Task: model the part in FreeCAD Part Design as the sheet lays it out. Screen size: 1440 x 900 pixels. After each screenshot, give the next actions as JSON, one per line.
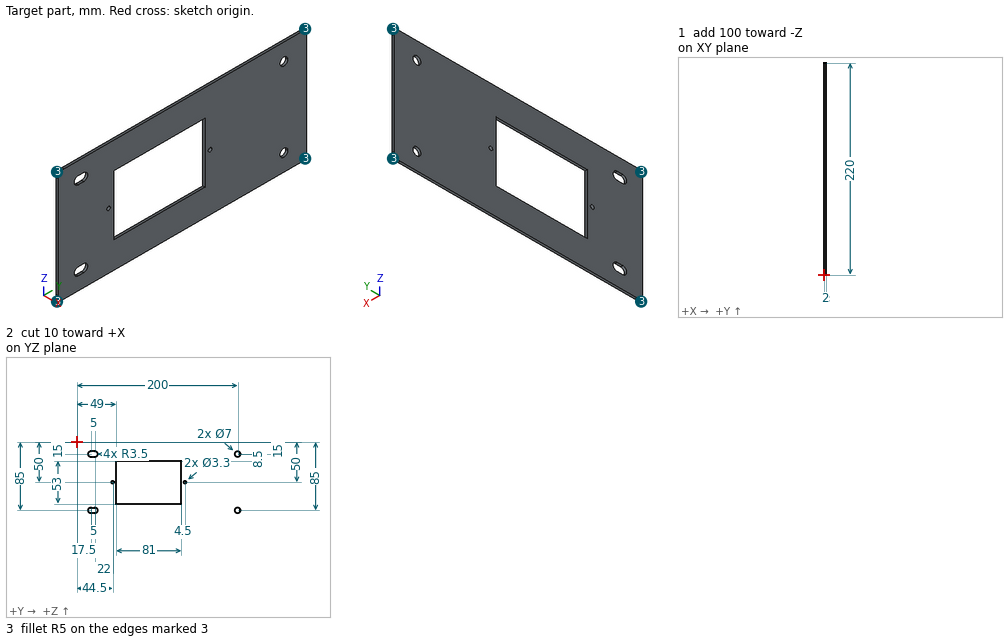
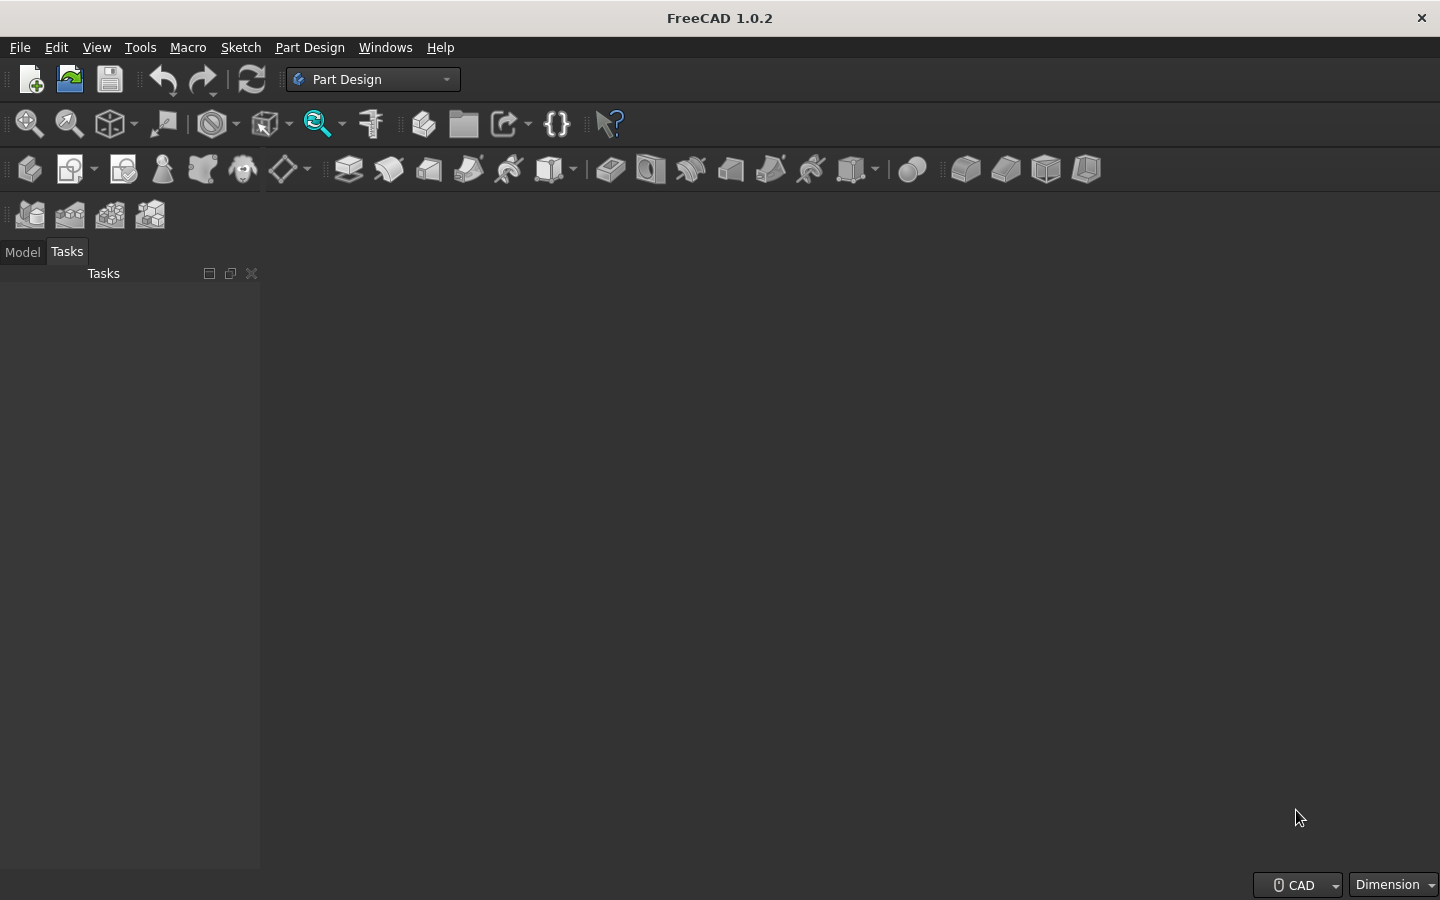
{"action": "left_click", "coordinate": [1024, 80]}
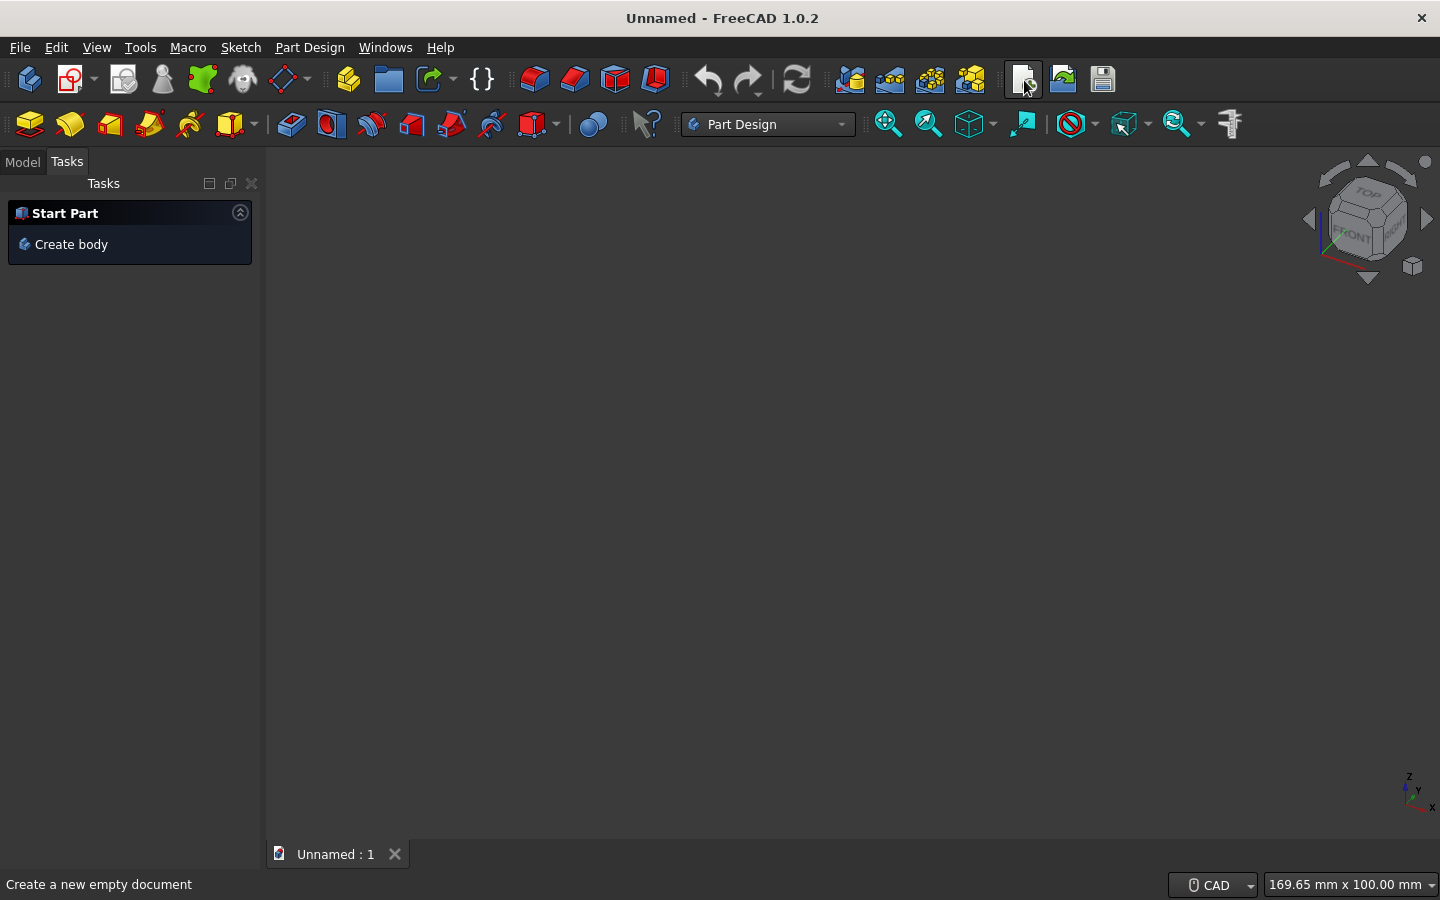
{"action": "left_click", "coordinate": [70, 80]}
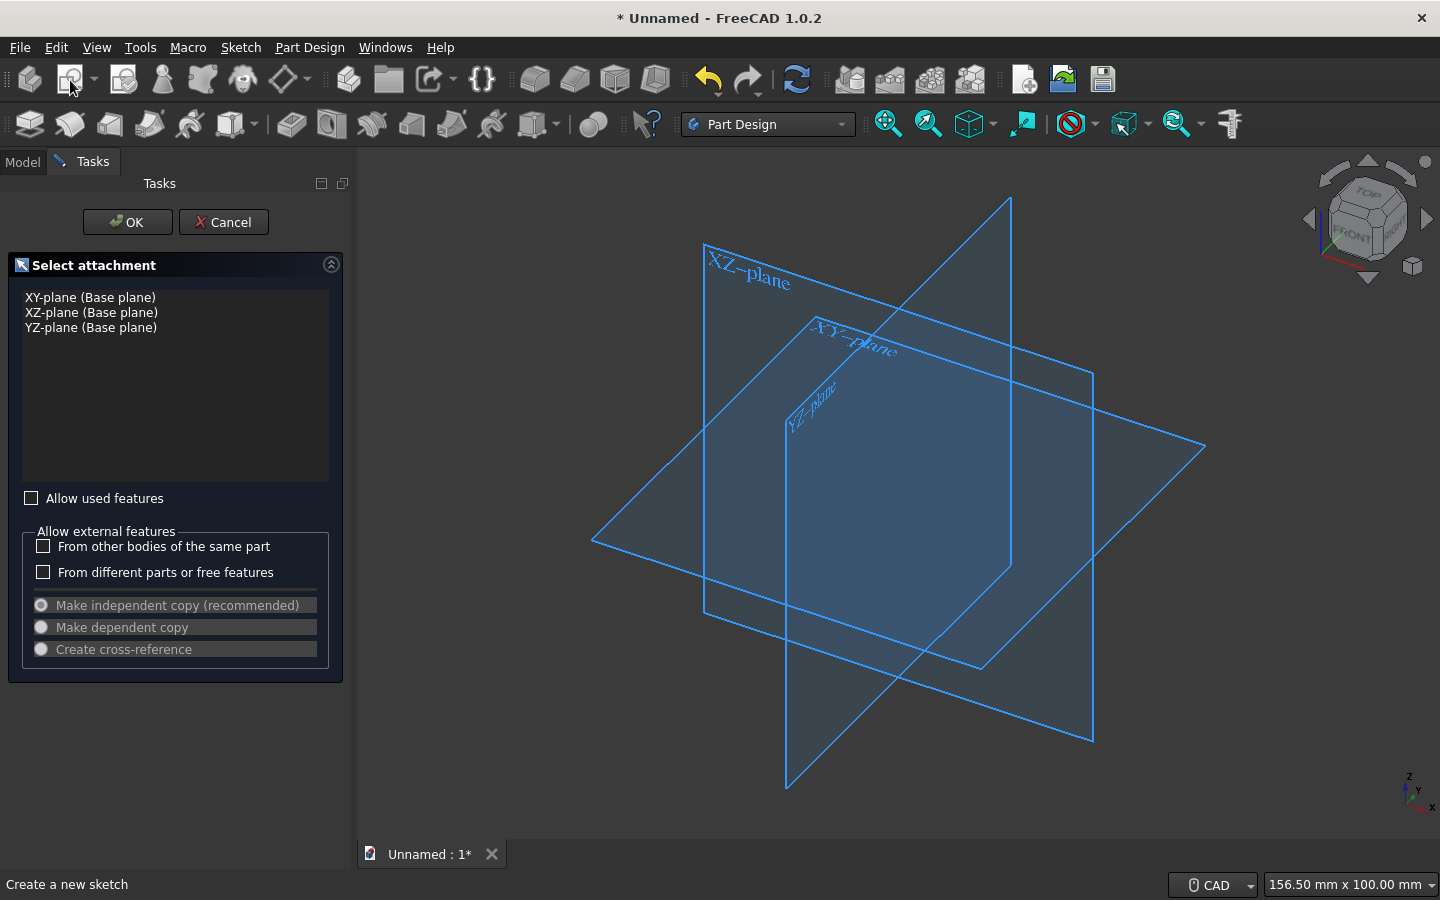
{"action": "left_click", "coordinate": [82, 298]}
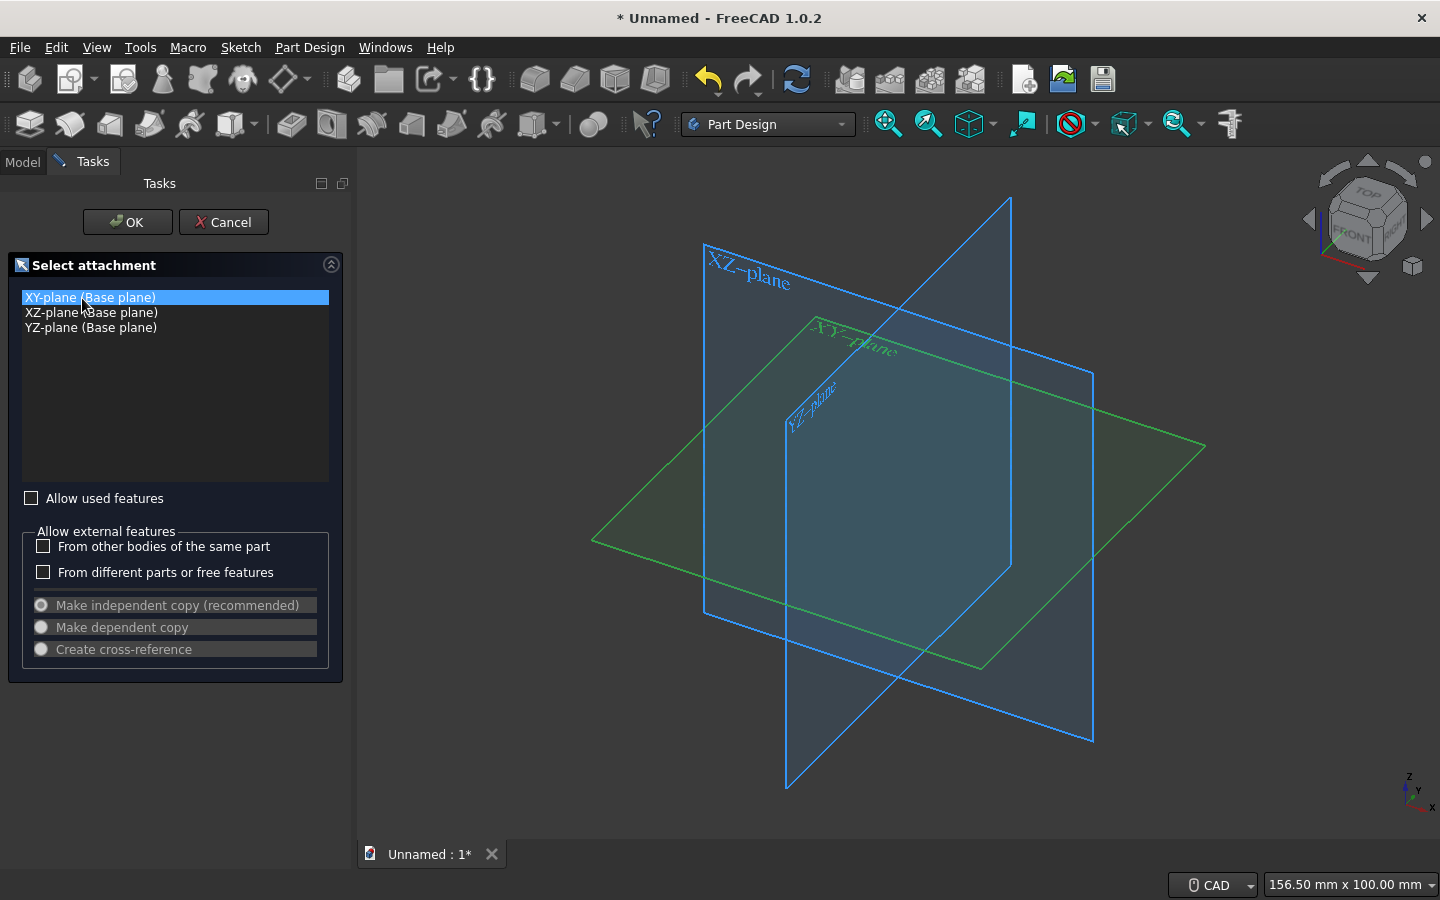
{"action": "left_click", "coordinate": [128, 222]}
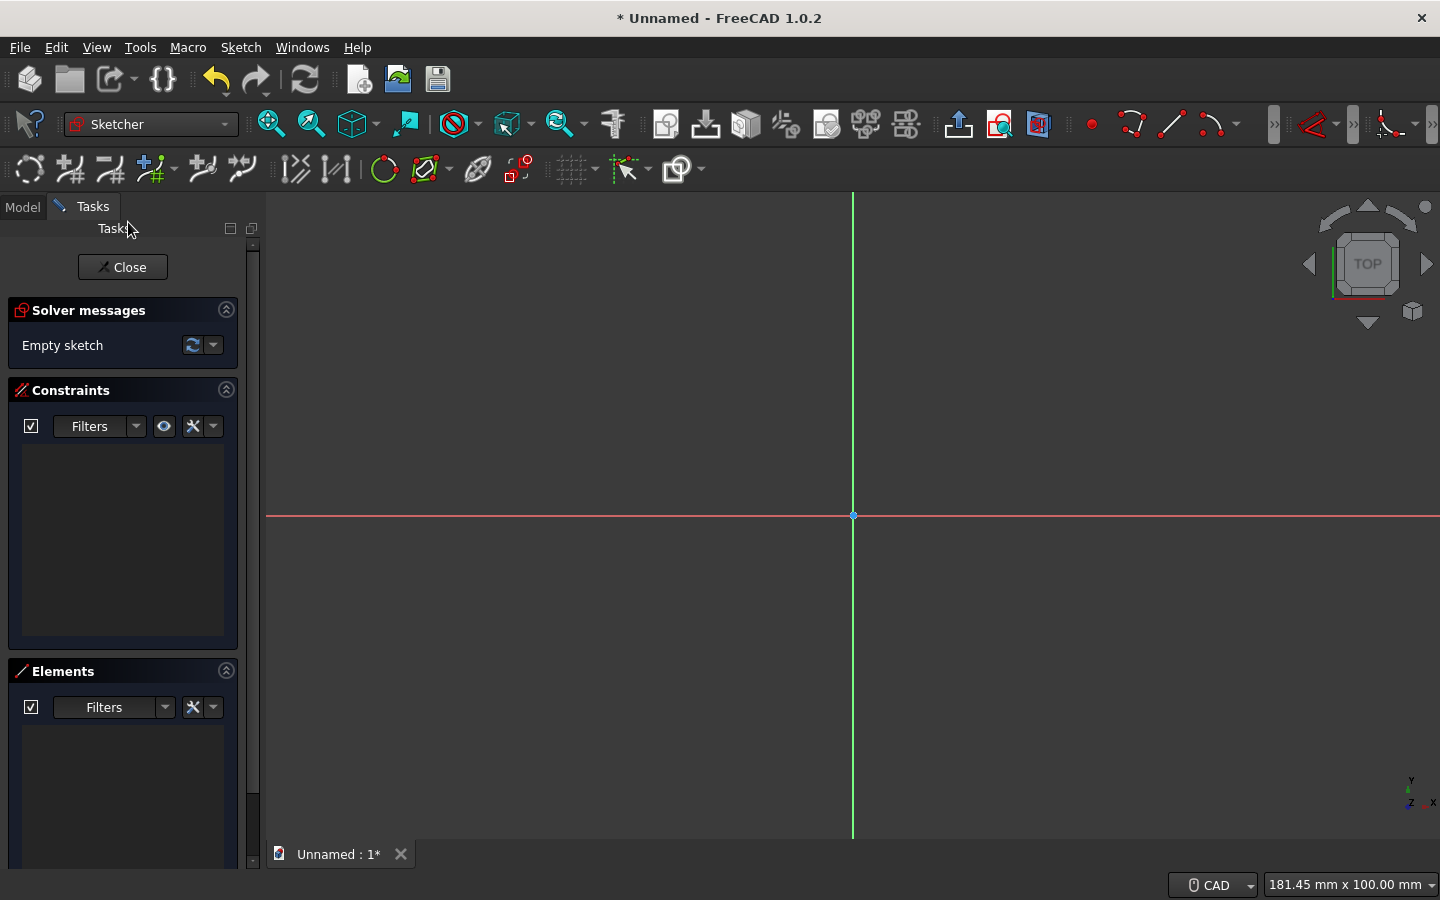
{"action": "scroll", "coordinate": [752, 811], "scroll_direction": "down", "scroll_amount": 6}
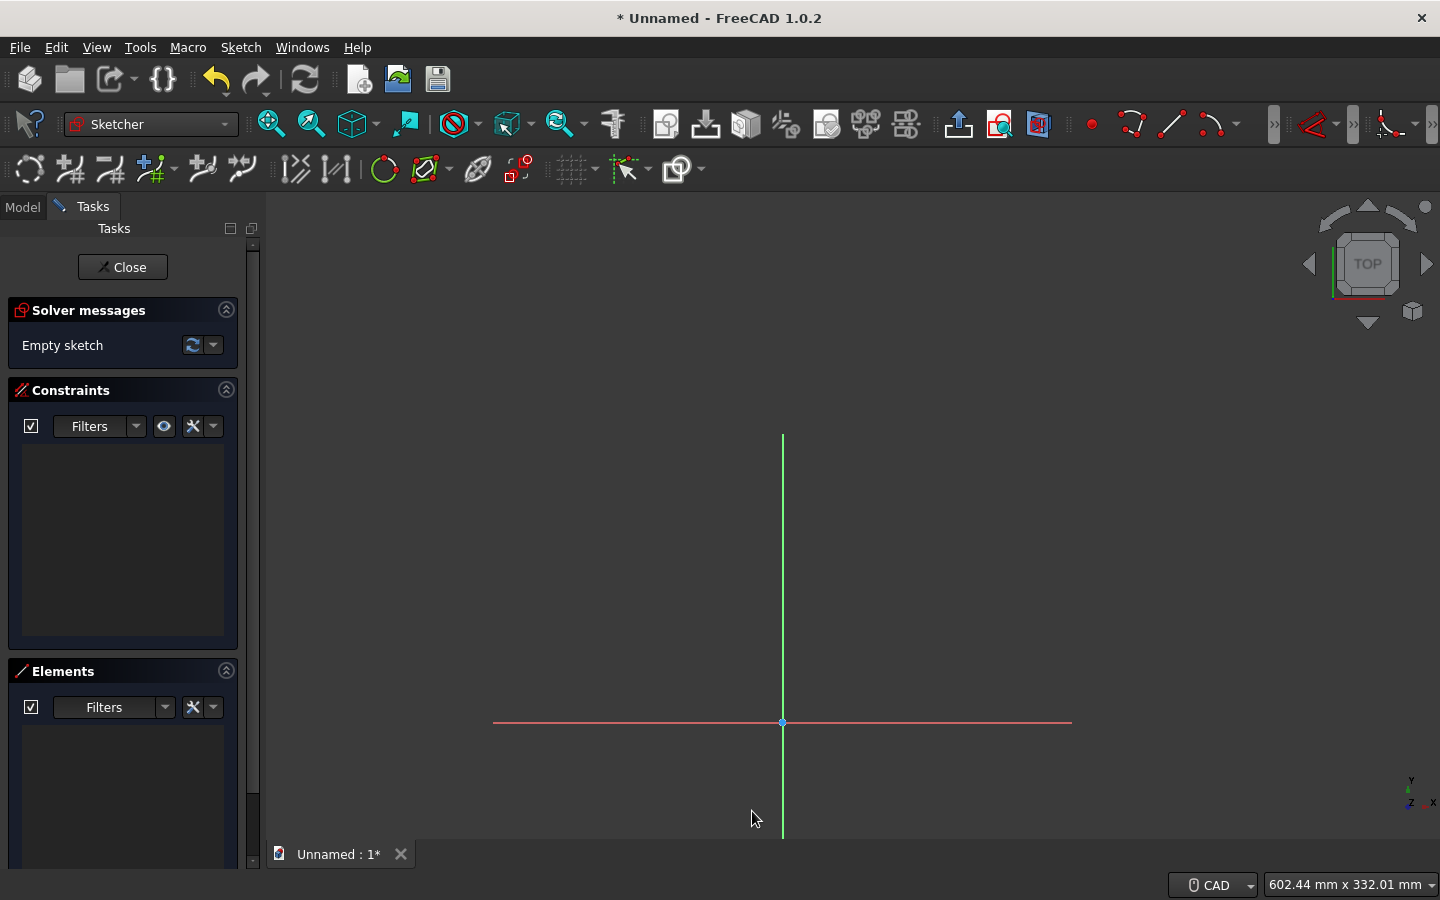
{"action": "key", "text": "g r"}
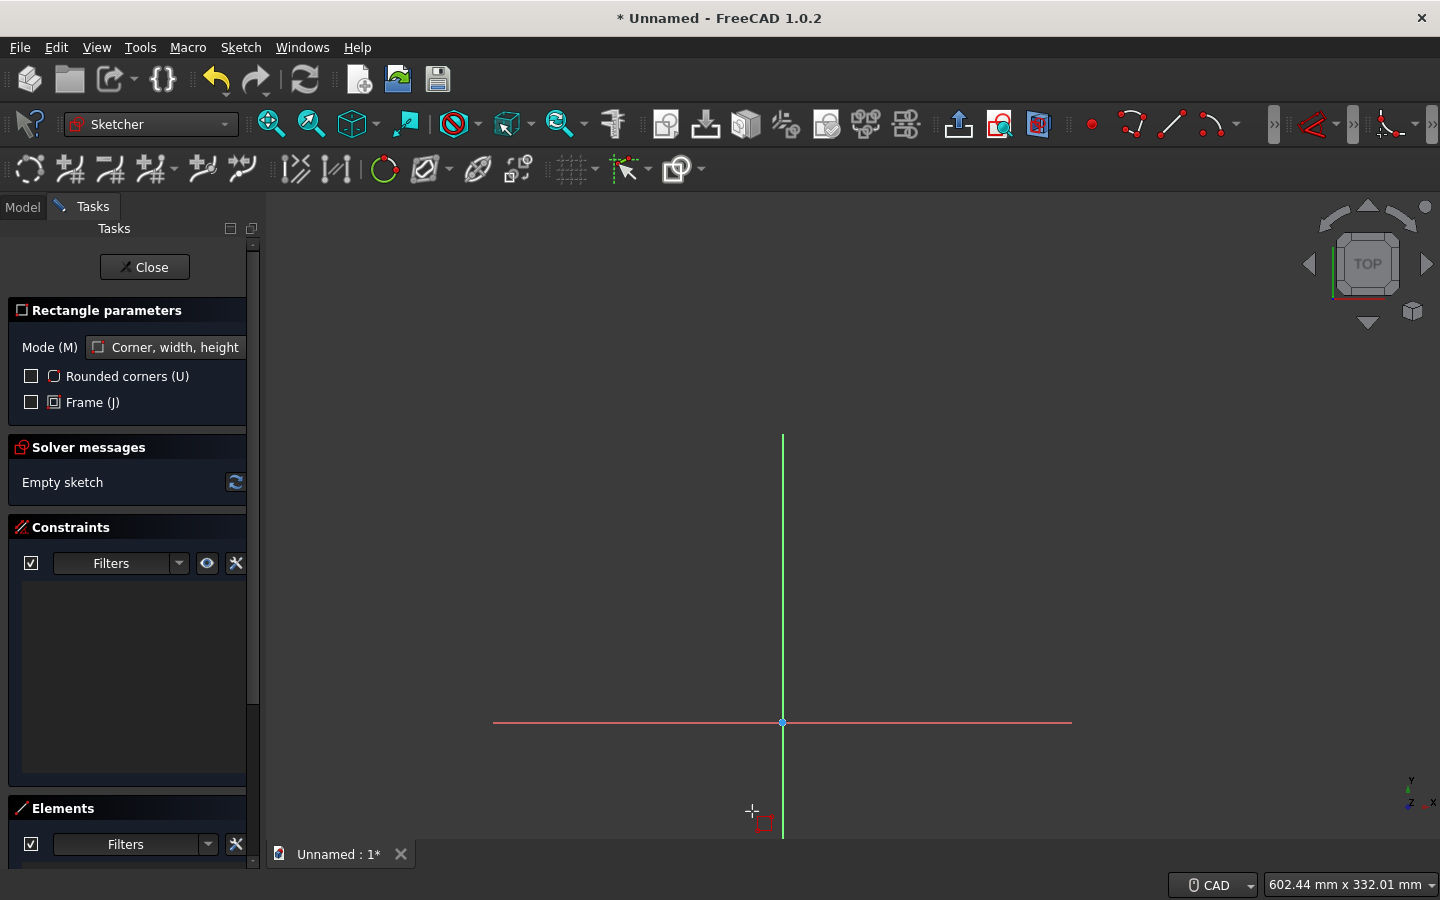
{"action": "scroll", "coordinate": [783, 723], "scroll_direction": "up", "scroll_amount": 8}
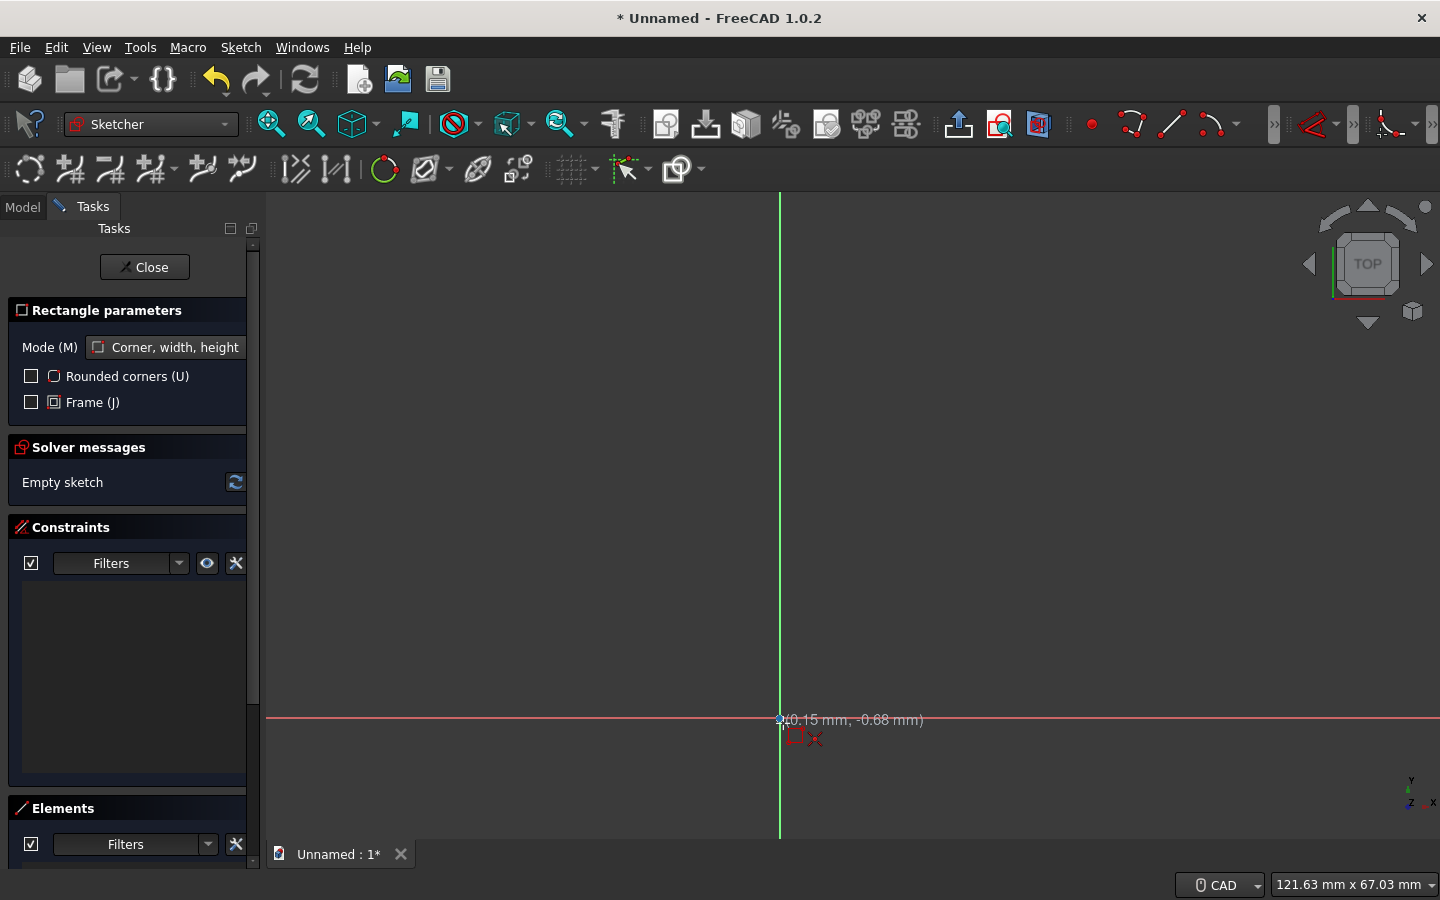
{"action": "scroll", "coordinate": [783, 733], "scroll_direction": "down", "scroll_amount": 8}